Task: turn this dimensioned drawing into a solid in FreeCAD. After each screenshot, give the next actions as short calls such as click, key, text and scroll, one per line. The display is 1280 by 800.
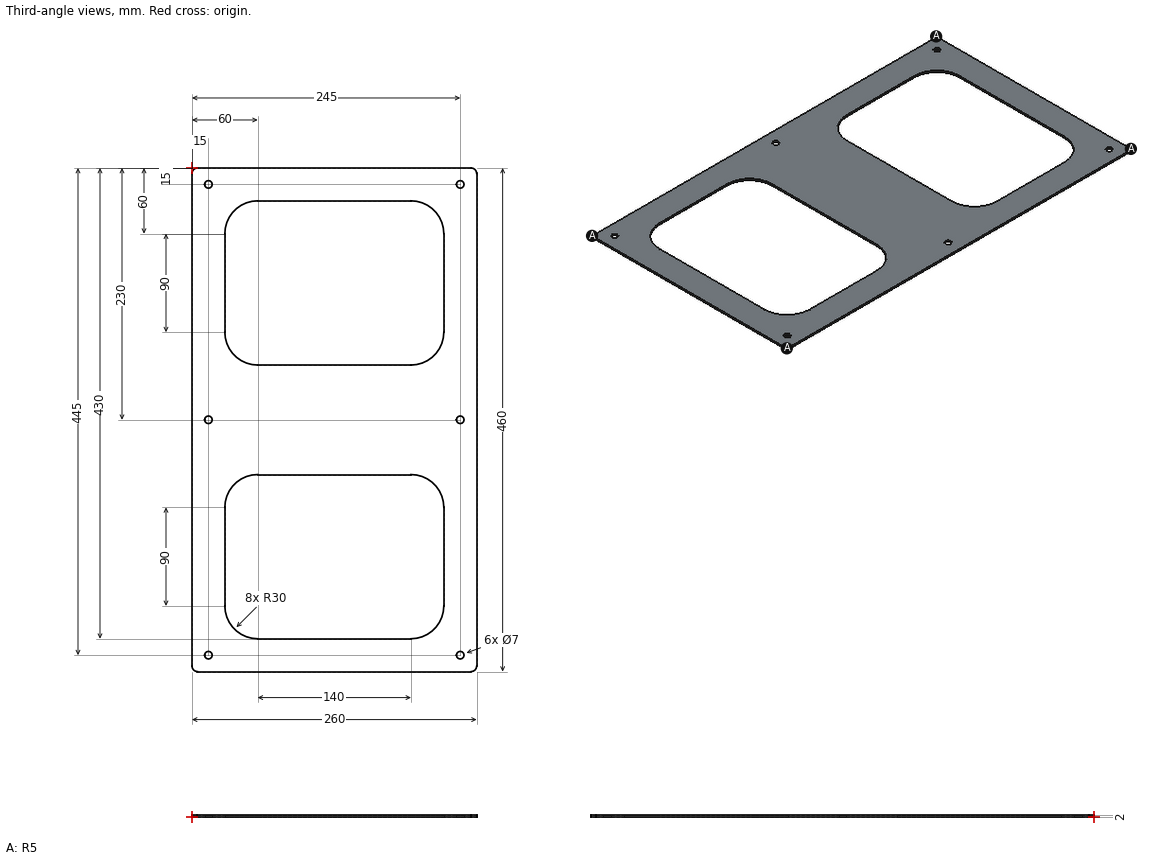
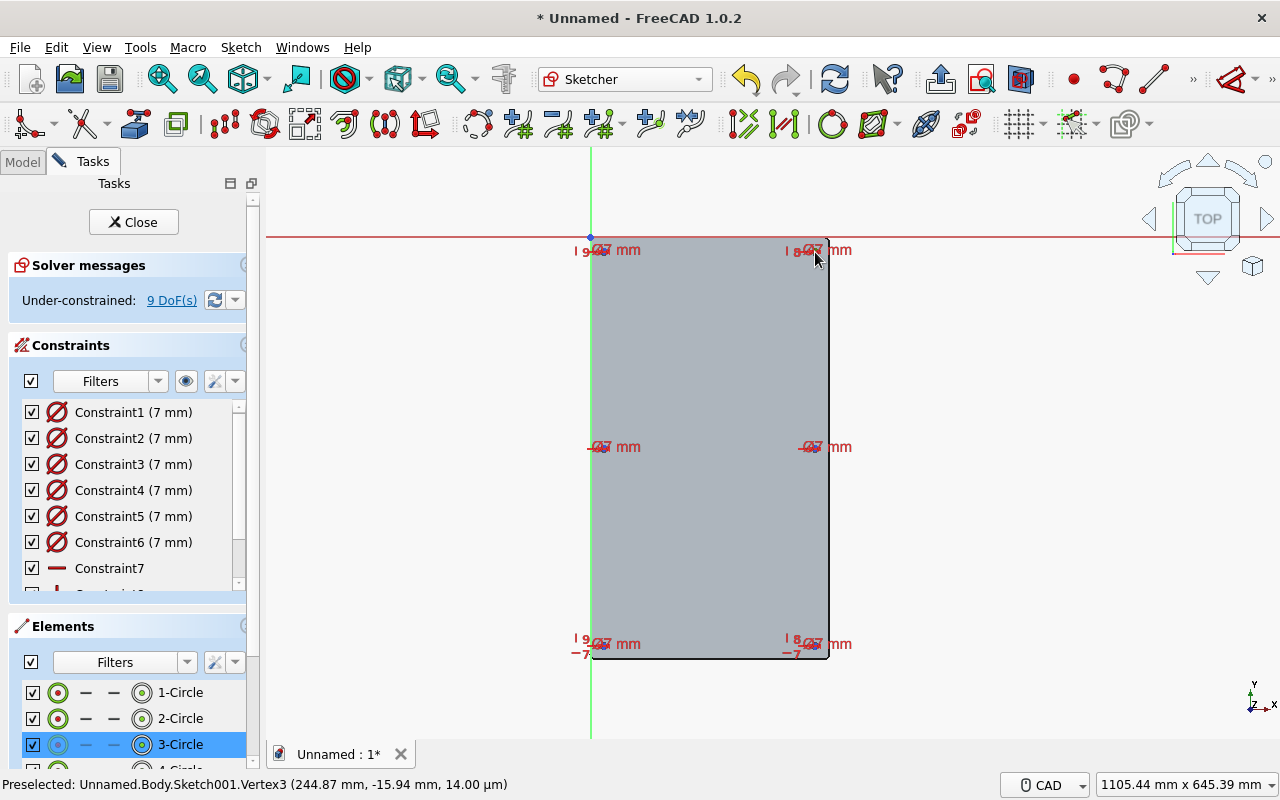
click(604, 252)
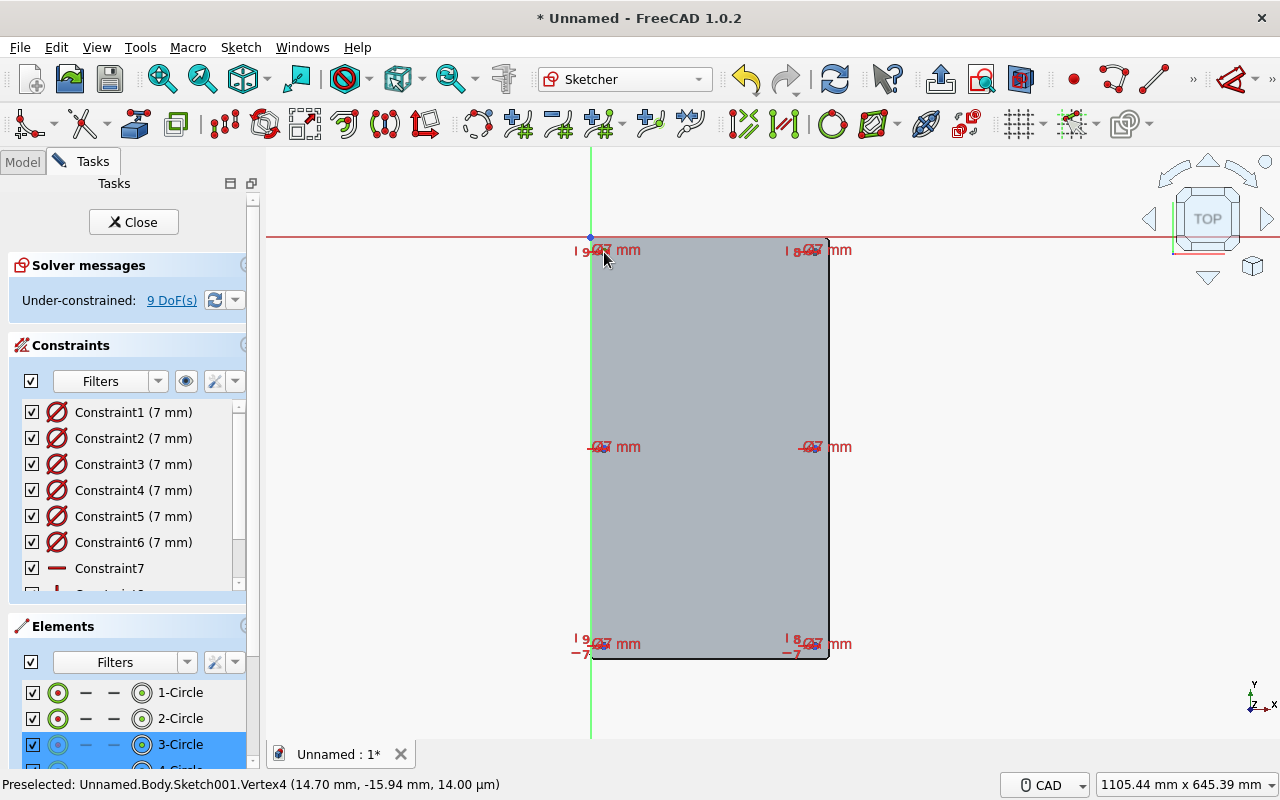
key(h)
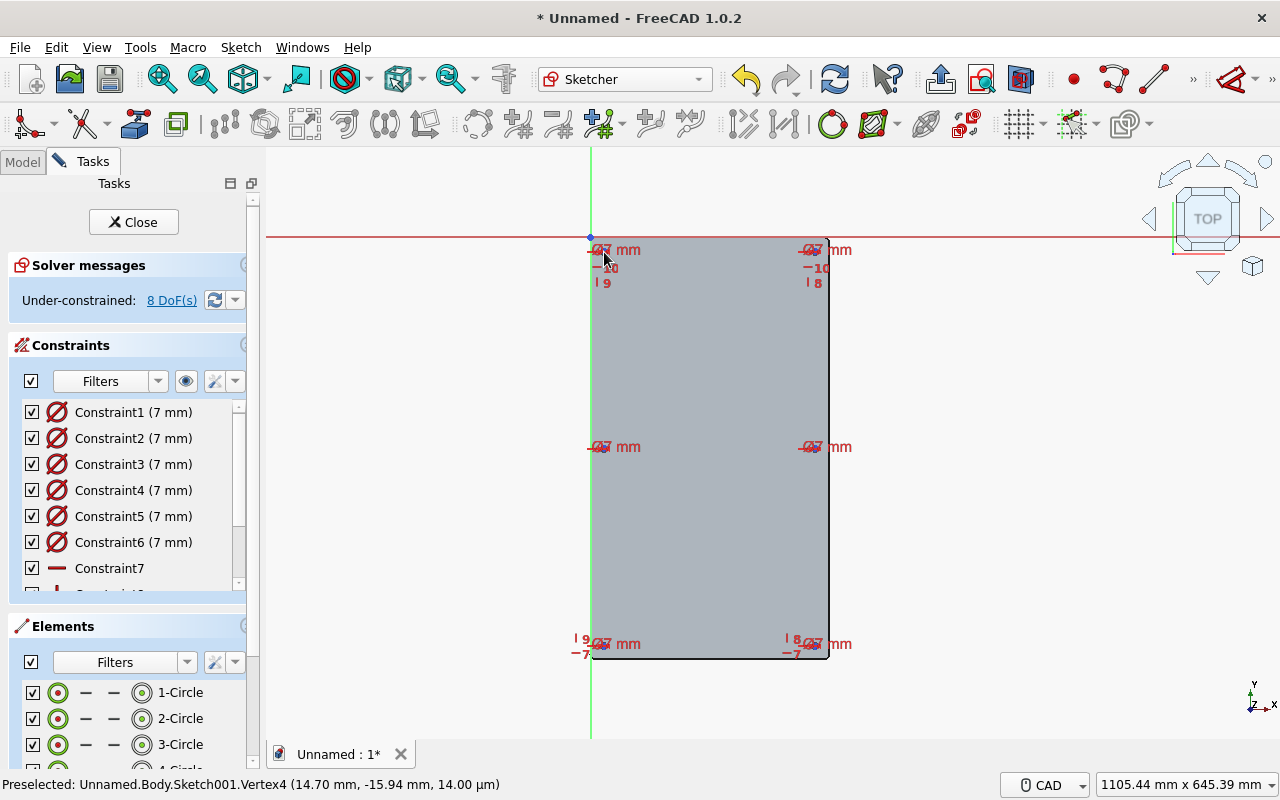
click(815, 646)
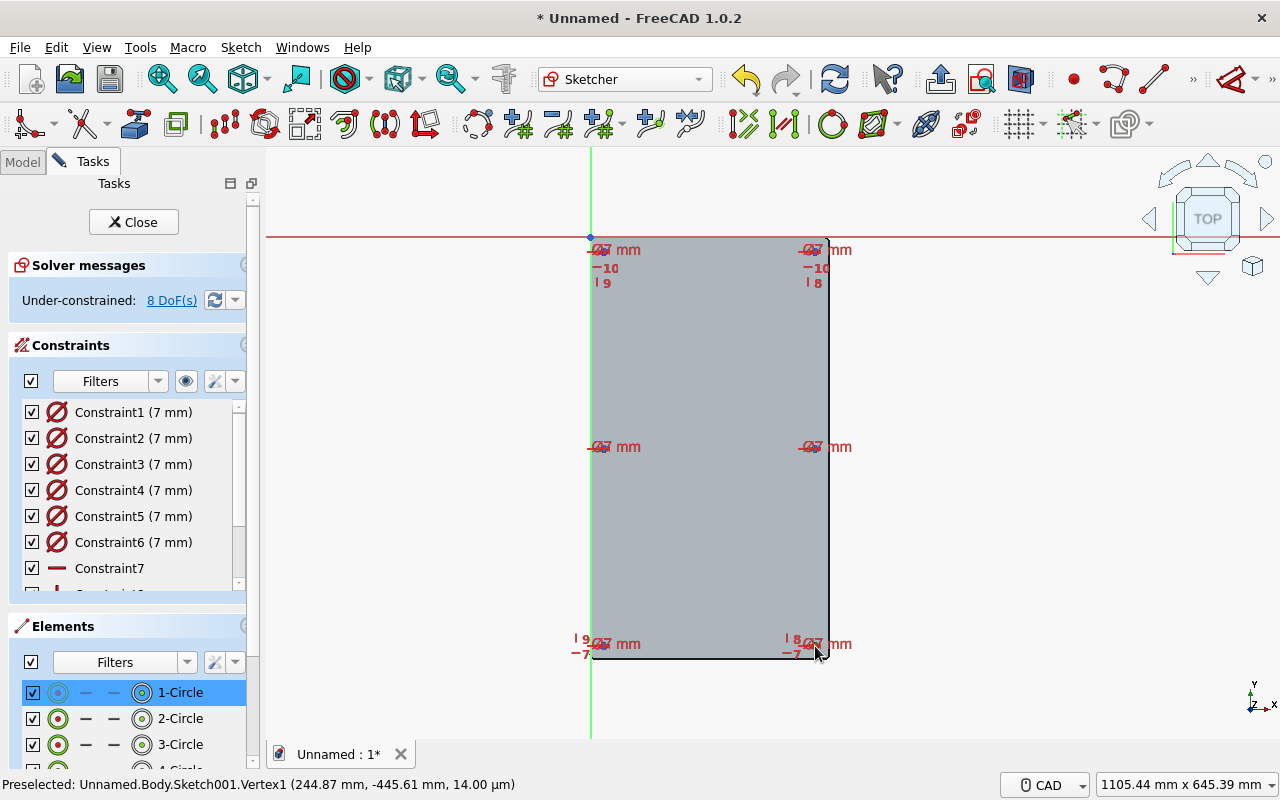
click(815, 449)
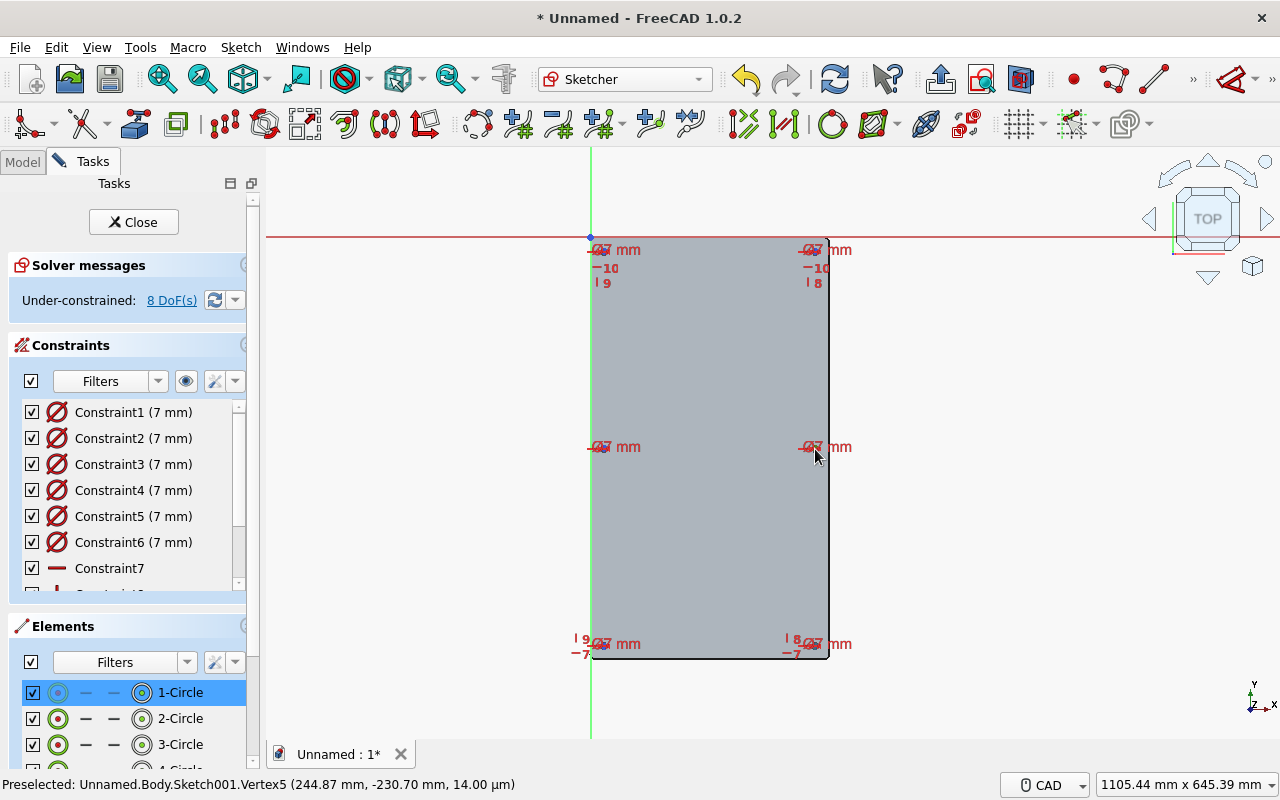
key(v)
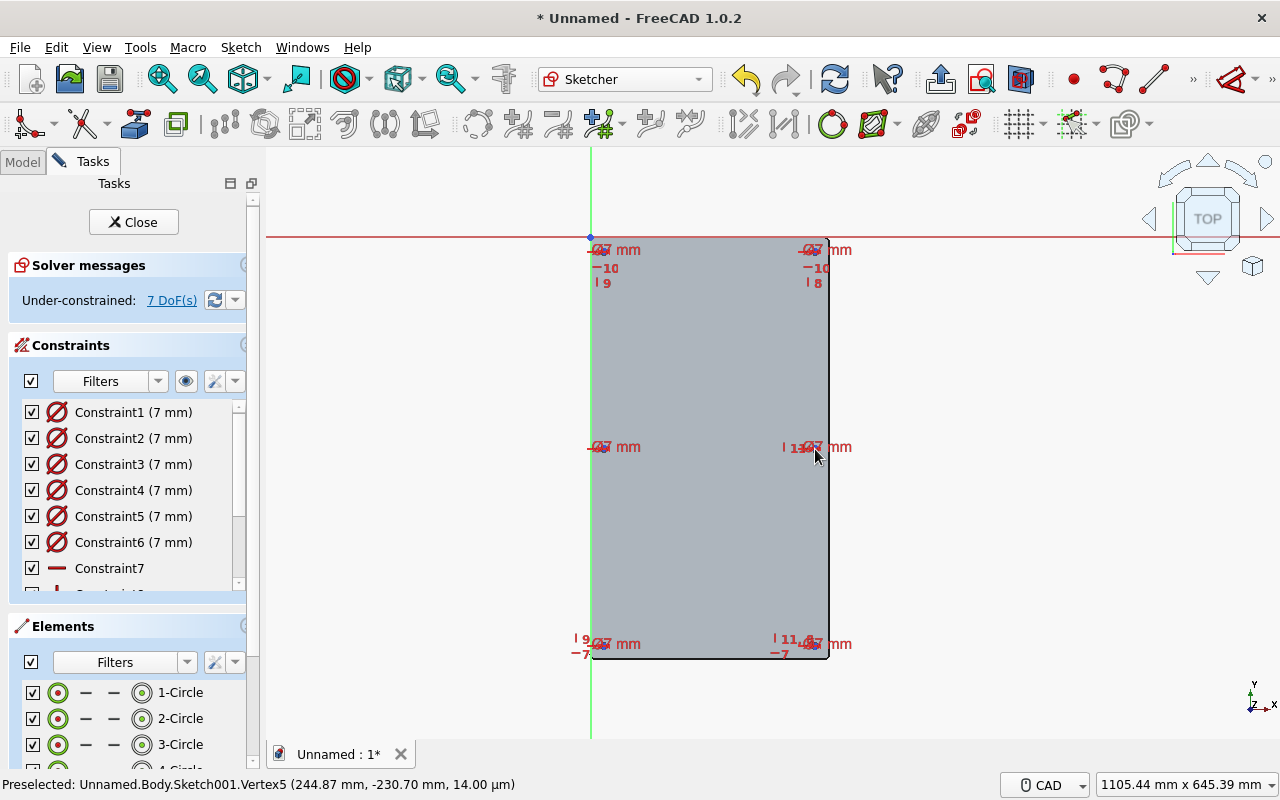
click(604, 646)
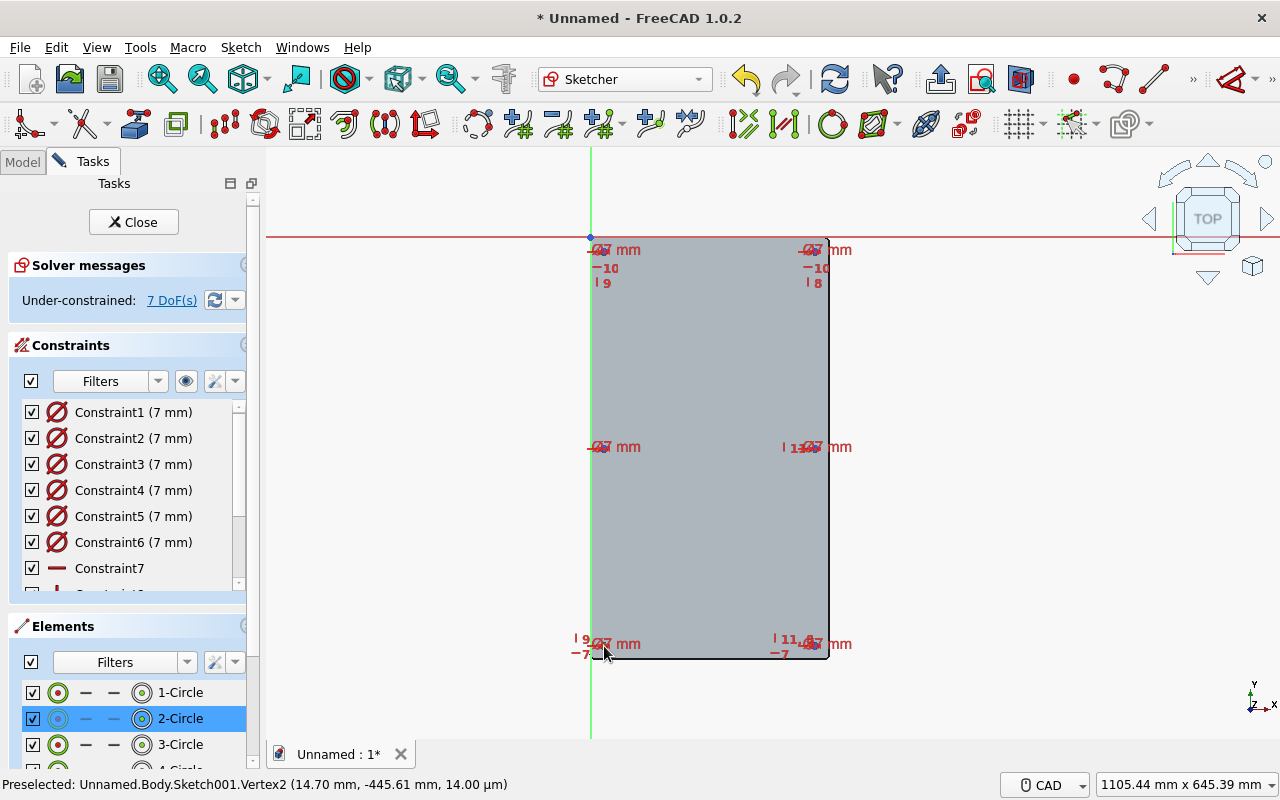
click(604, 449)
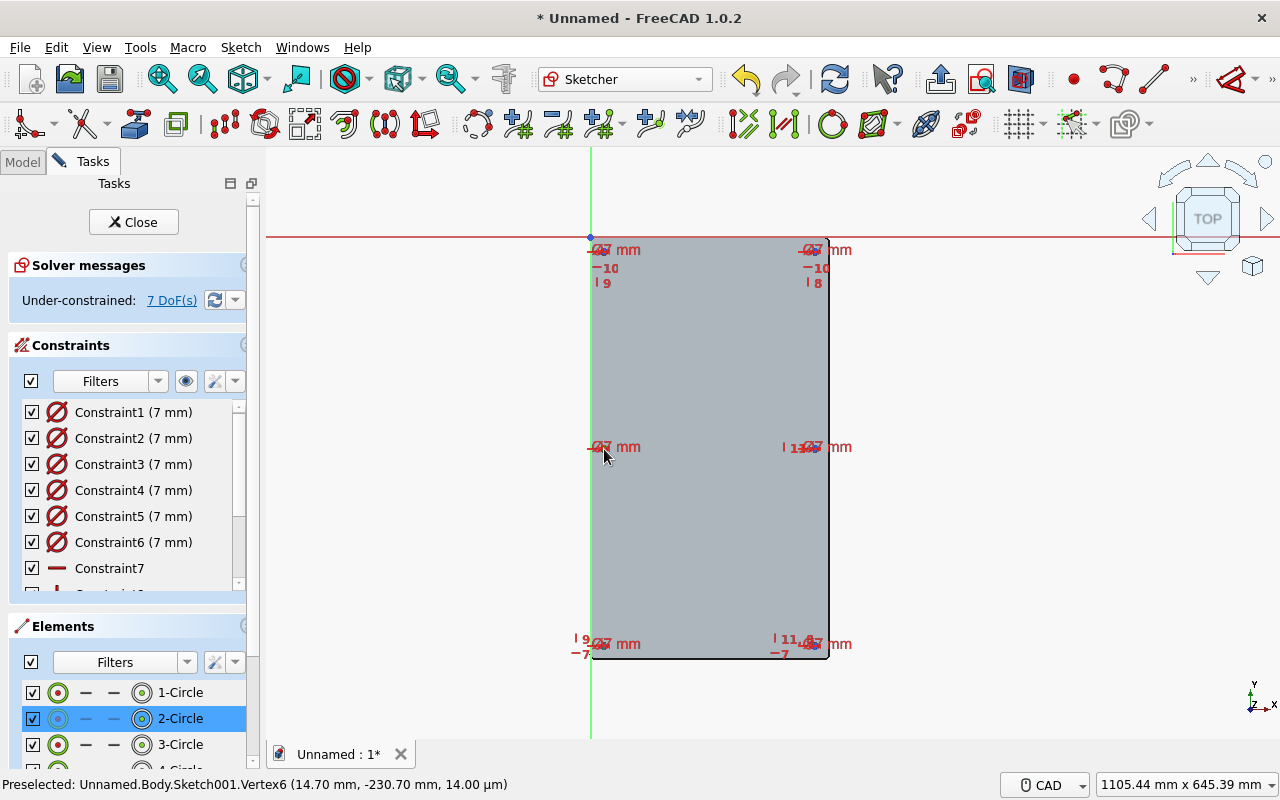
key(v)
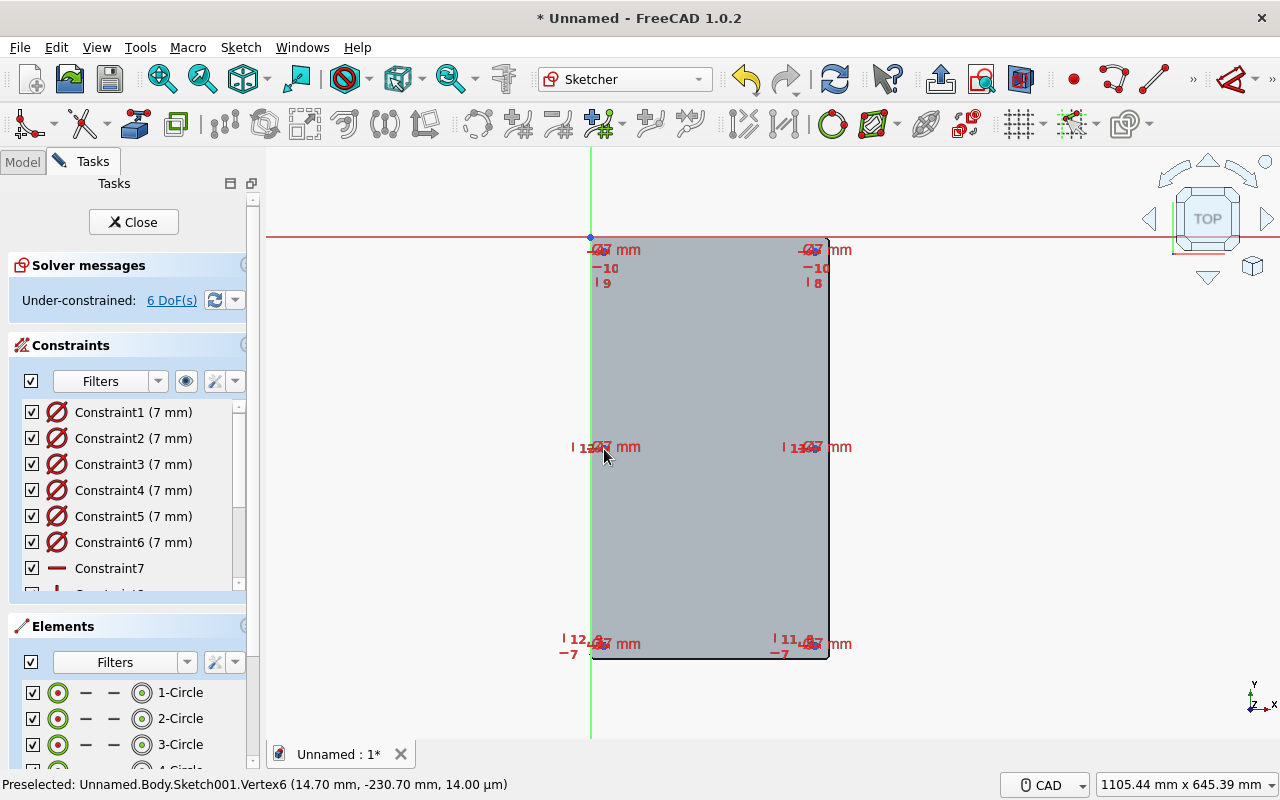
click(815, 449)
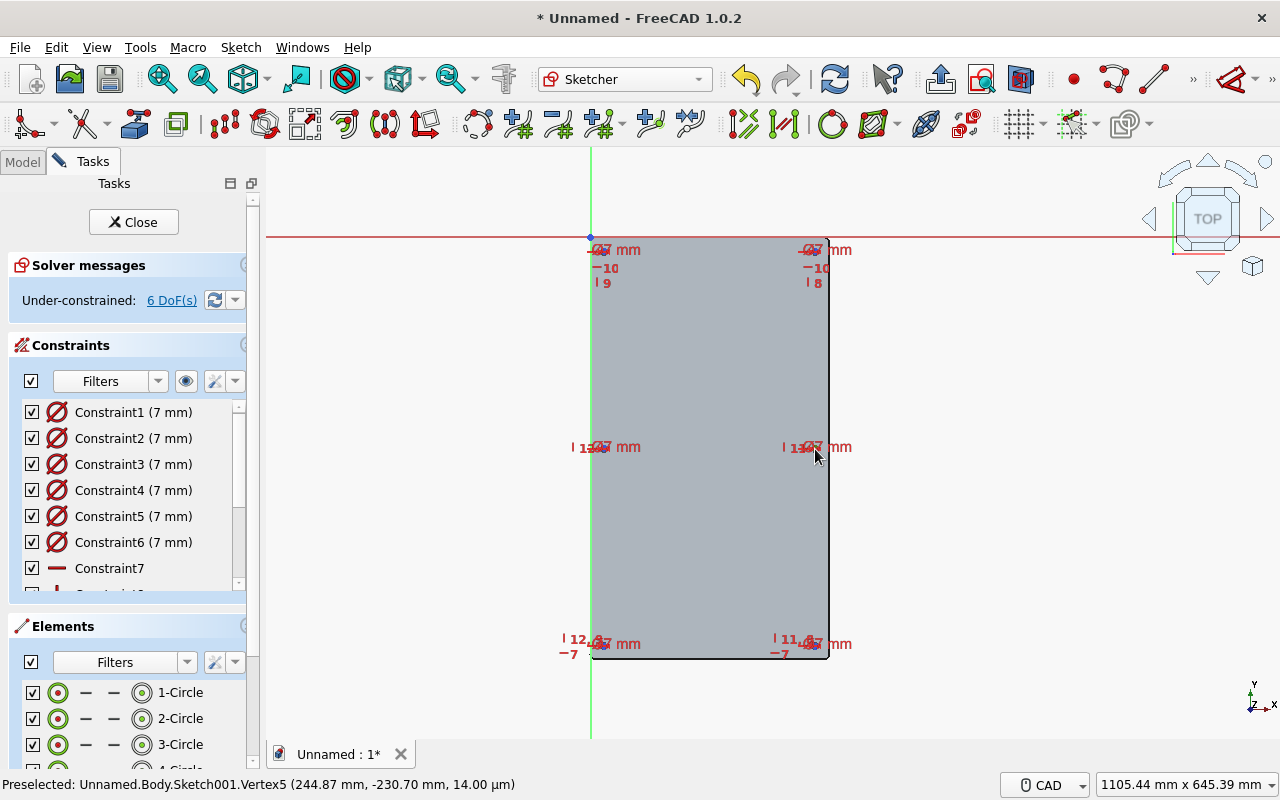
click(604, 449)